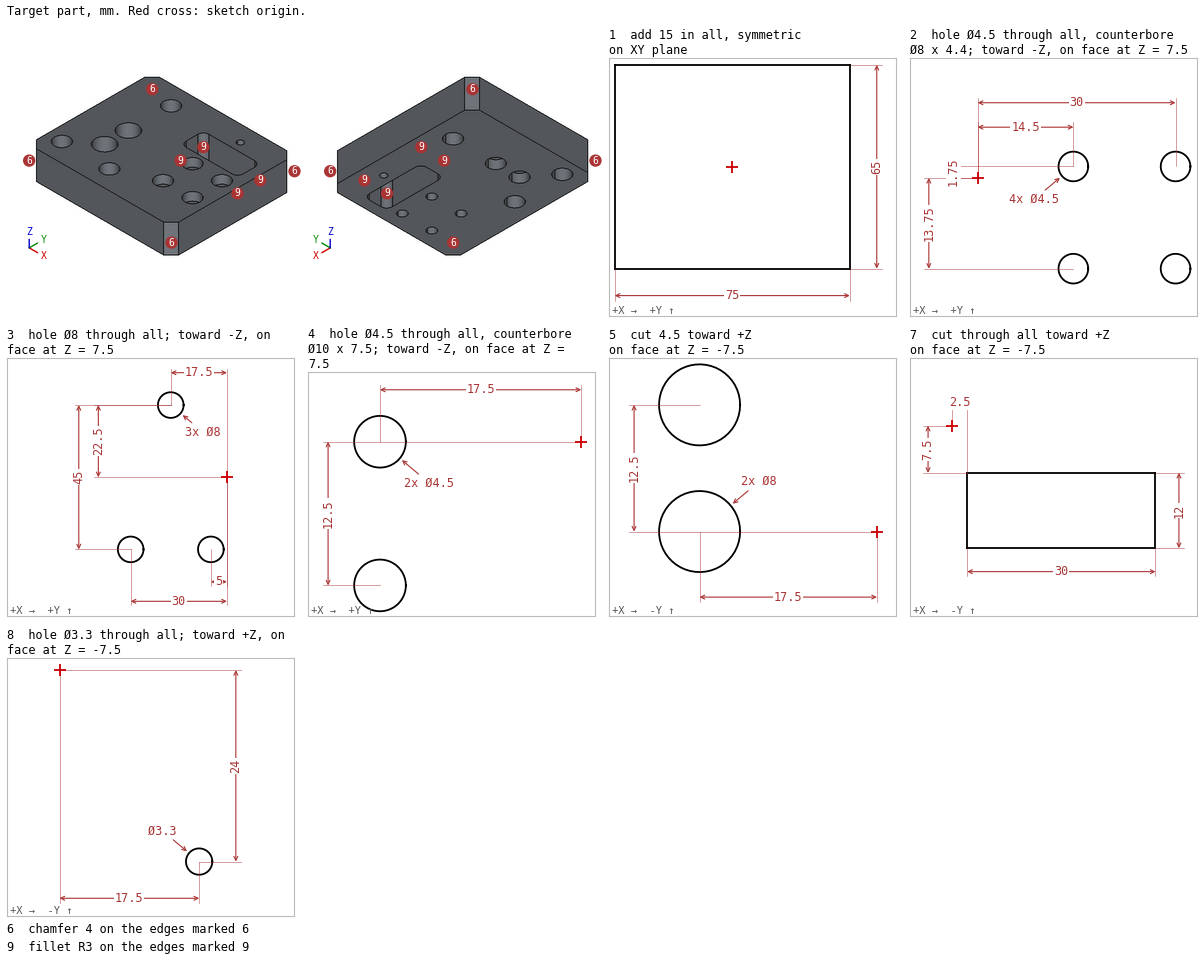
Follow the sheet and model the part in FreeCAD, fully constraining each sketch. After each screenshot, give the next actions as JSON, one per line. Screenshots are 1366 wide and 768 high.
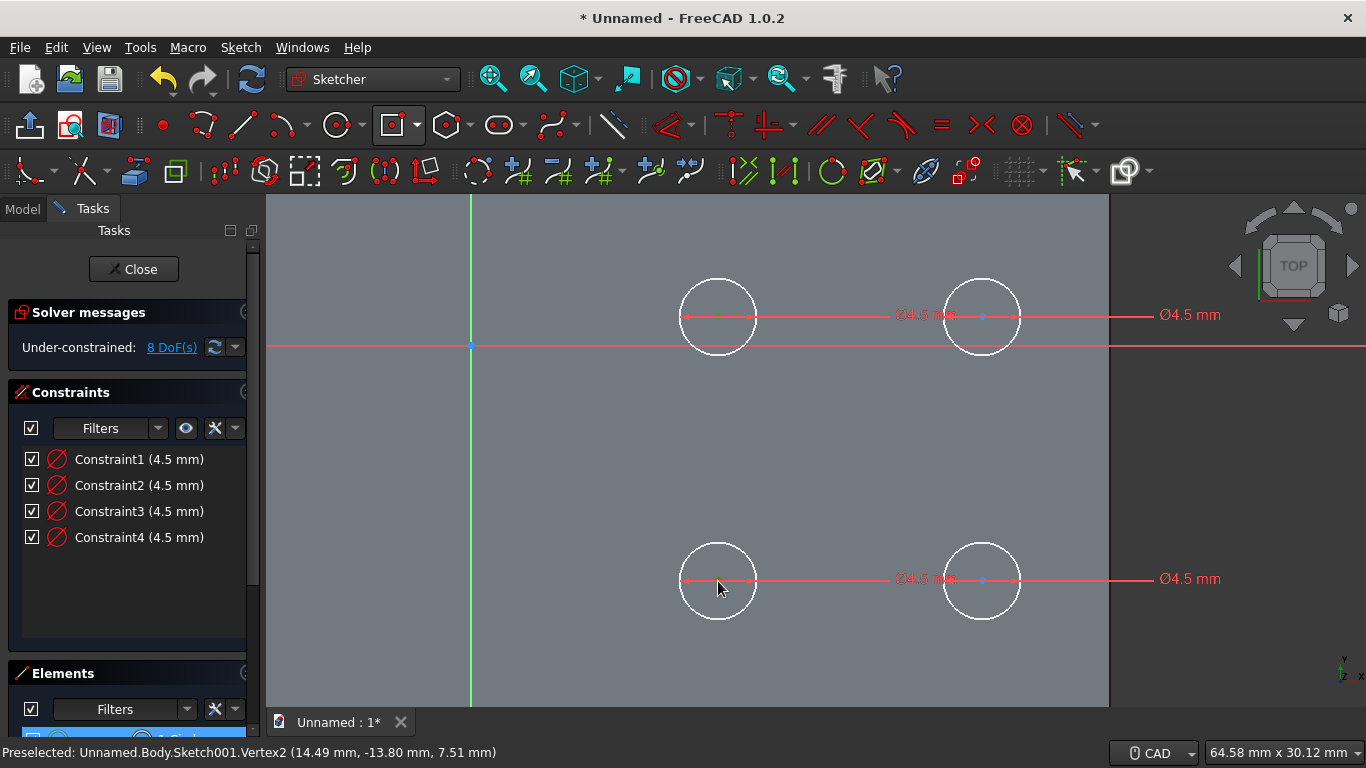
{"action": "left_click", "coordinate": [796, 126]}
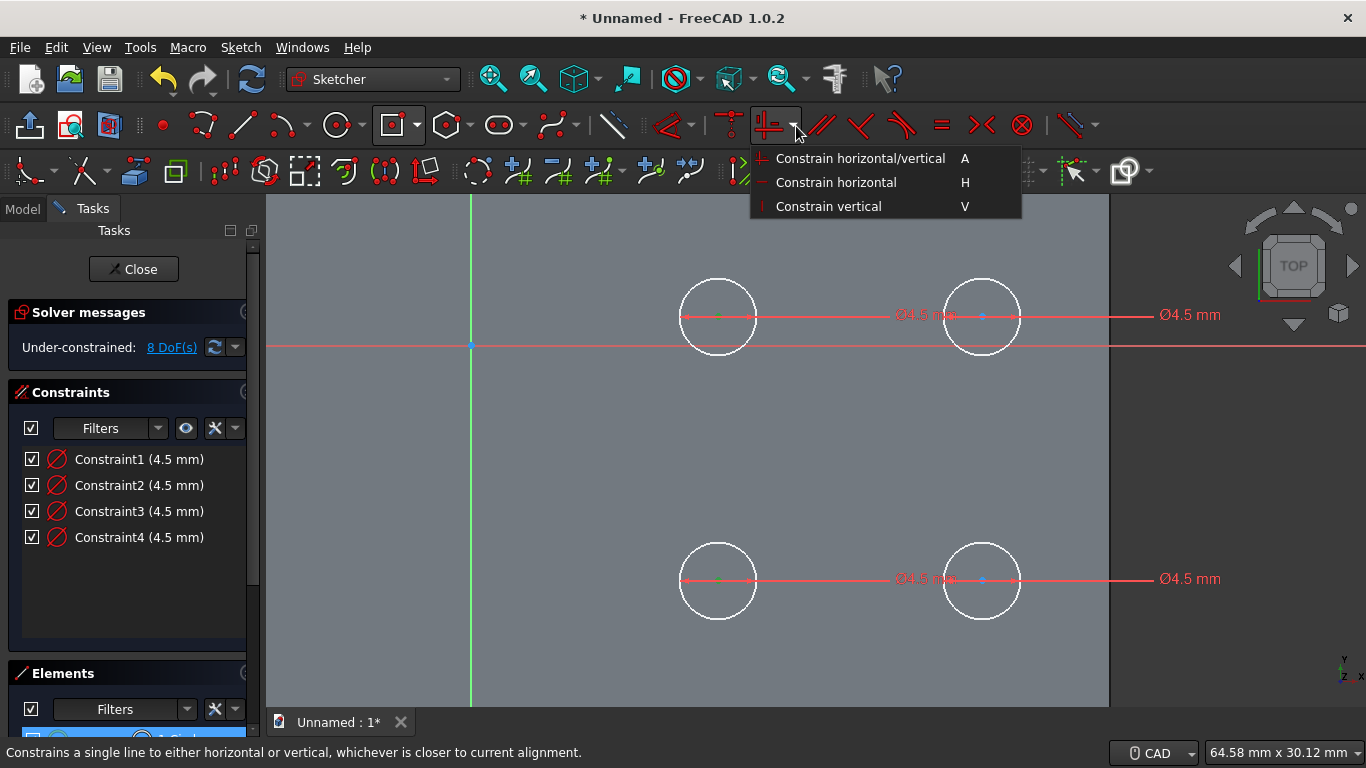
{"action": "left_click", "coordinate": [886, 206]}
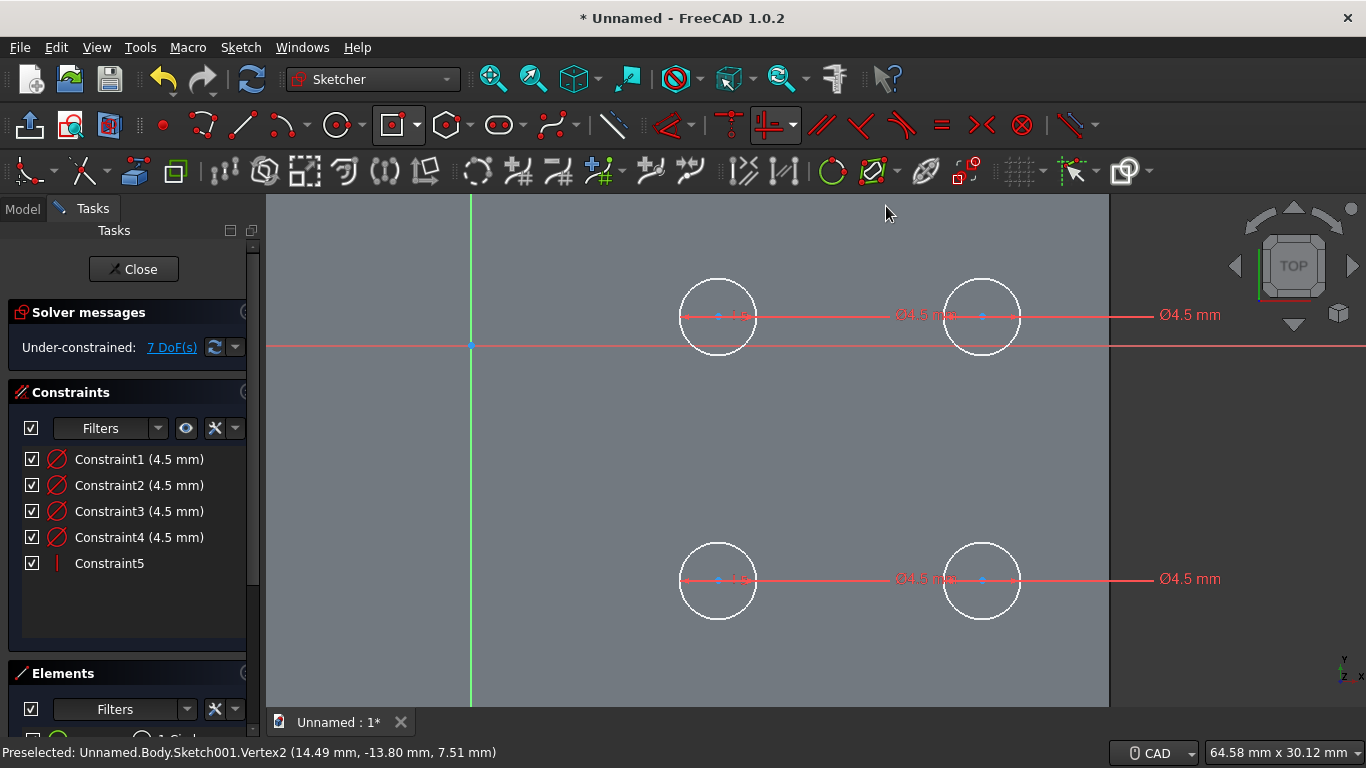
{"action": "left_click", "coordinate": [718, 317]}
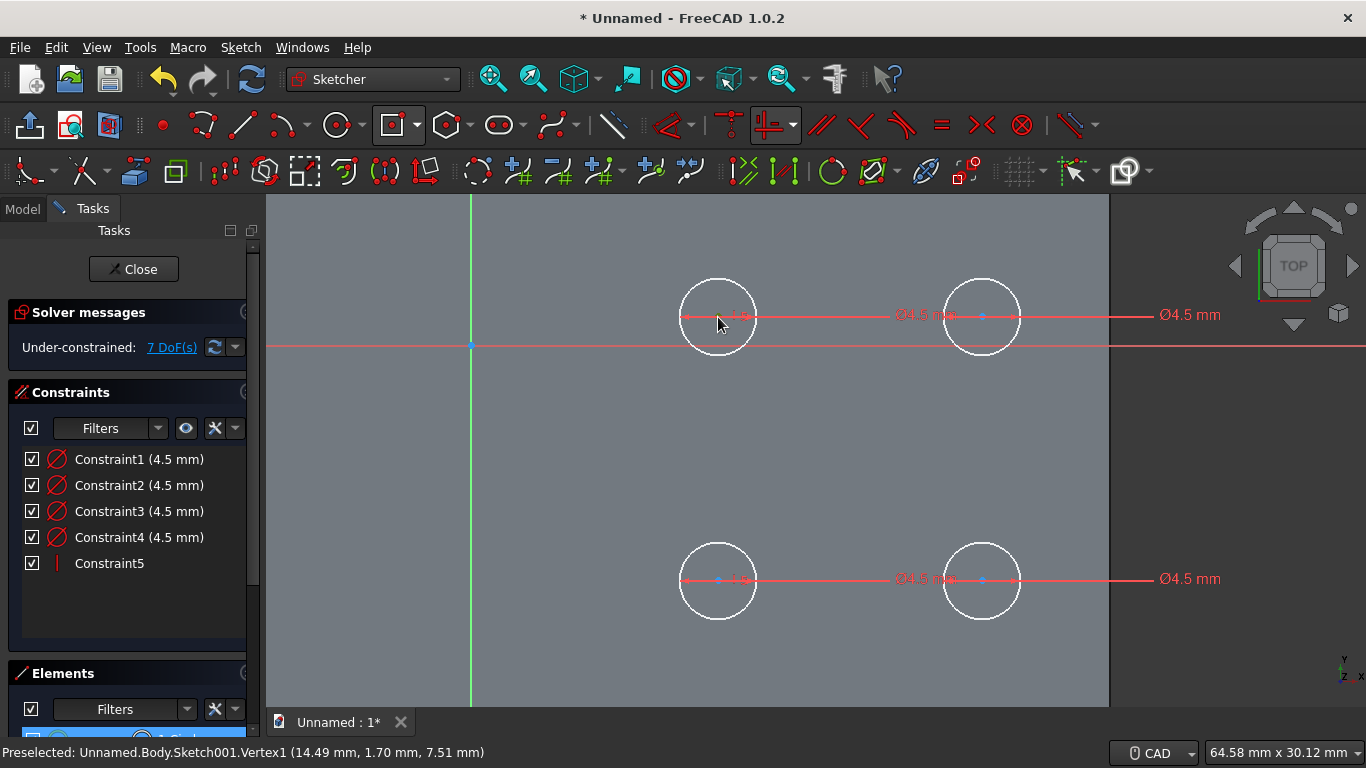
{"action": "left_click", "coordinate": [982, 317]}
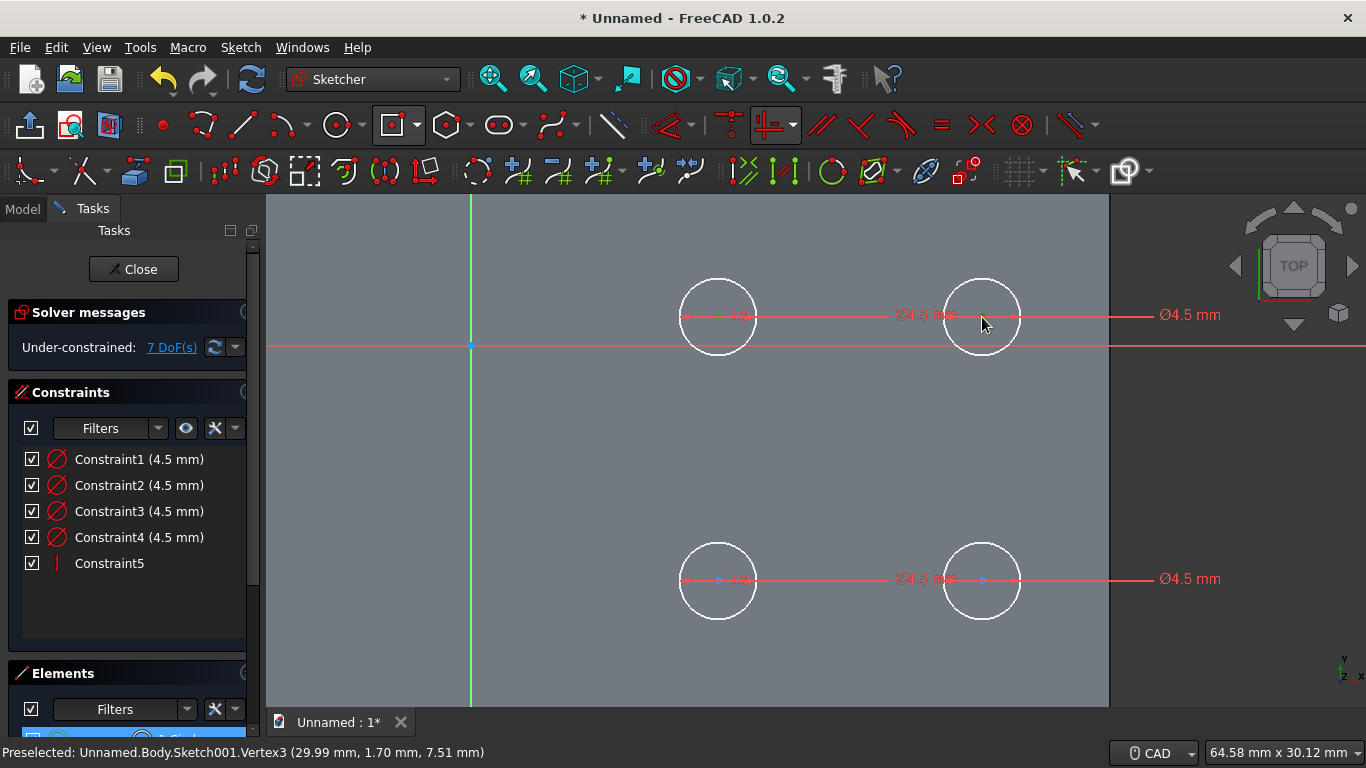
{"action": "left_click", "coordinate": [796, 126]}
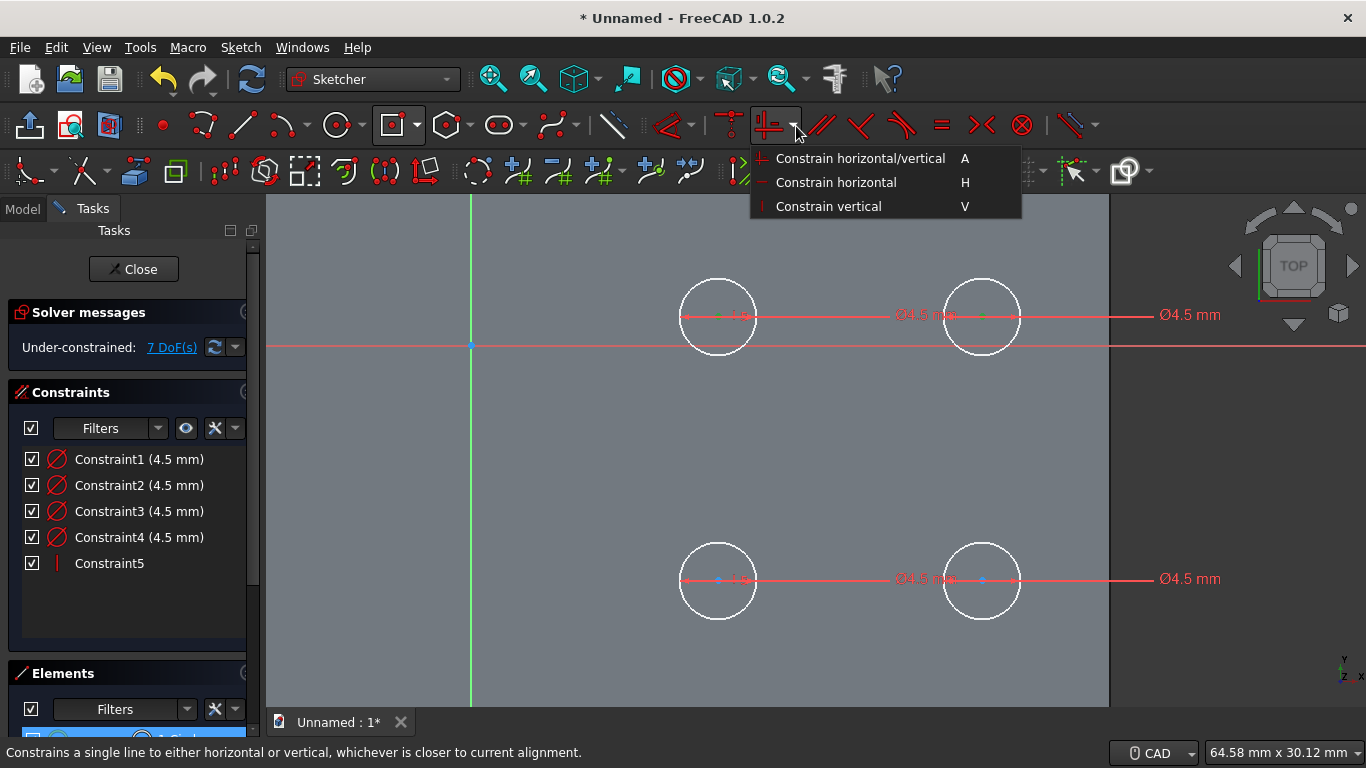
{"action": "left_click", "coordinate": [886, 182]}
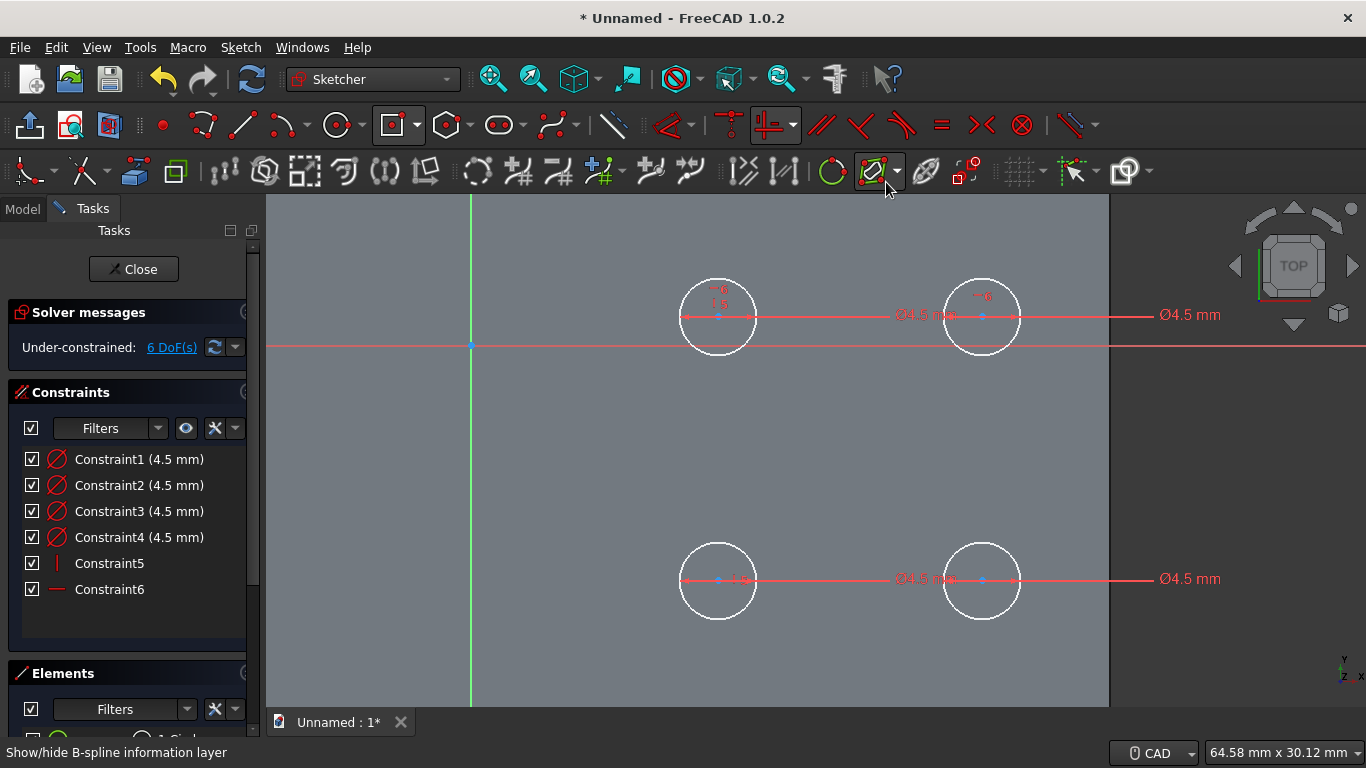
{"action": "left_click", "coordinate": [982, 317]}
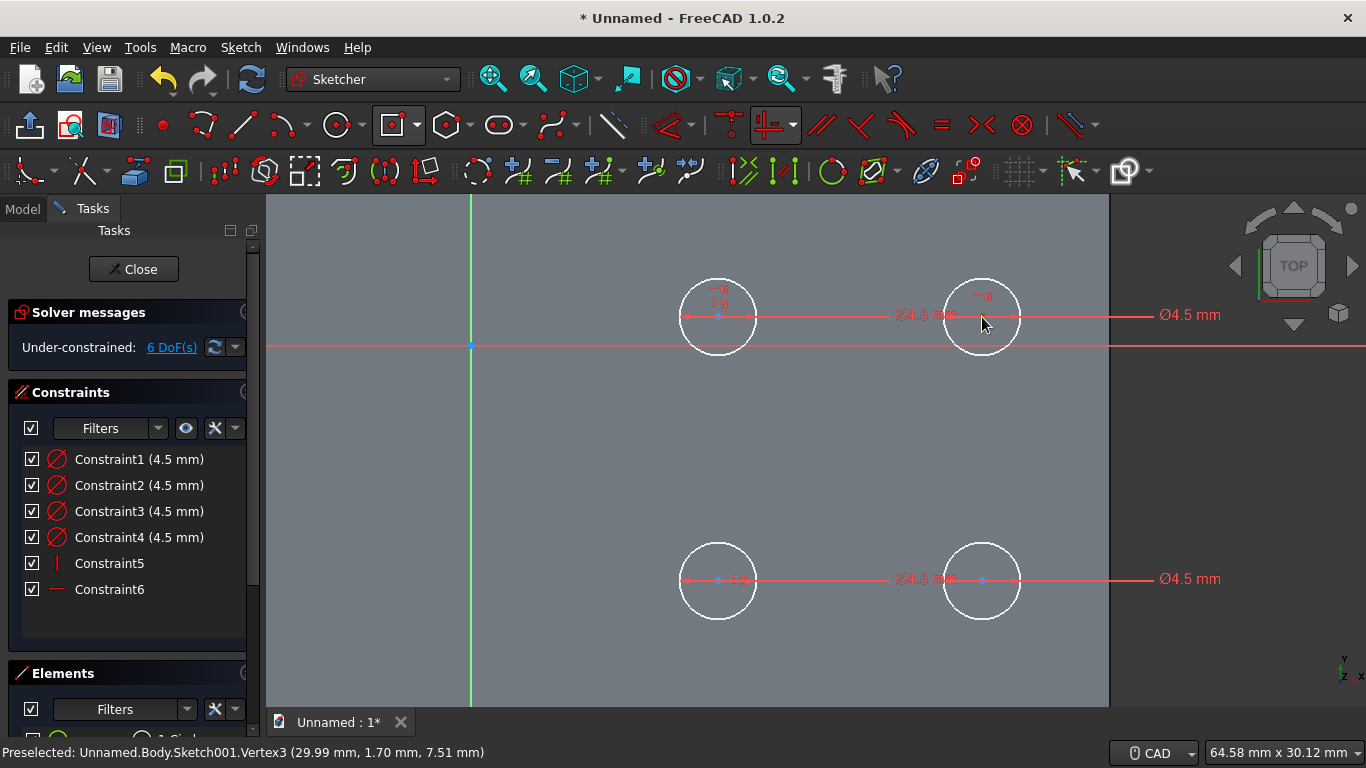
{"action": "left_click", "coordinate": [982, 581]}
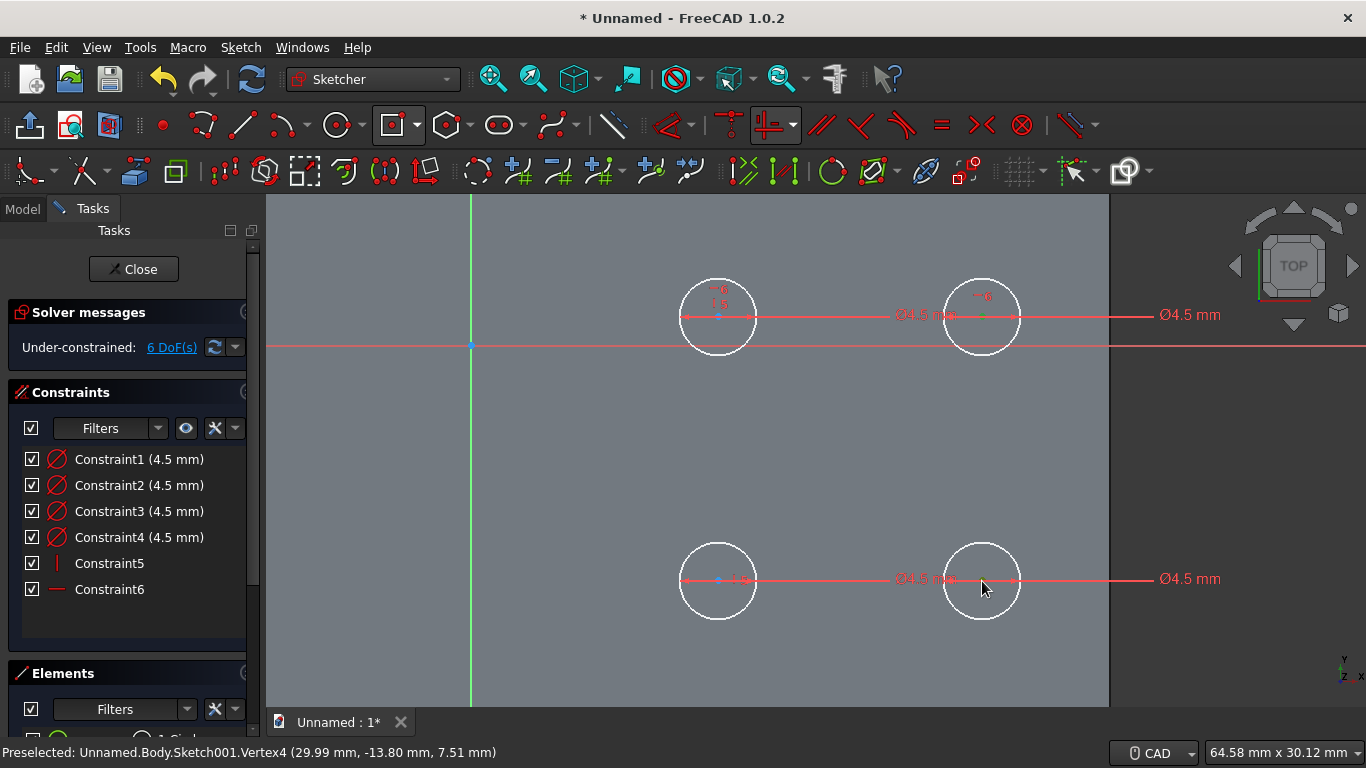
{"action": "left_click", "coordinate": [796, 126]}